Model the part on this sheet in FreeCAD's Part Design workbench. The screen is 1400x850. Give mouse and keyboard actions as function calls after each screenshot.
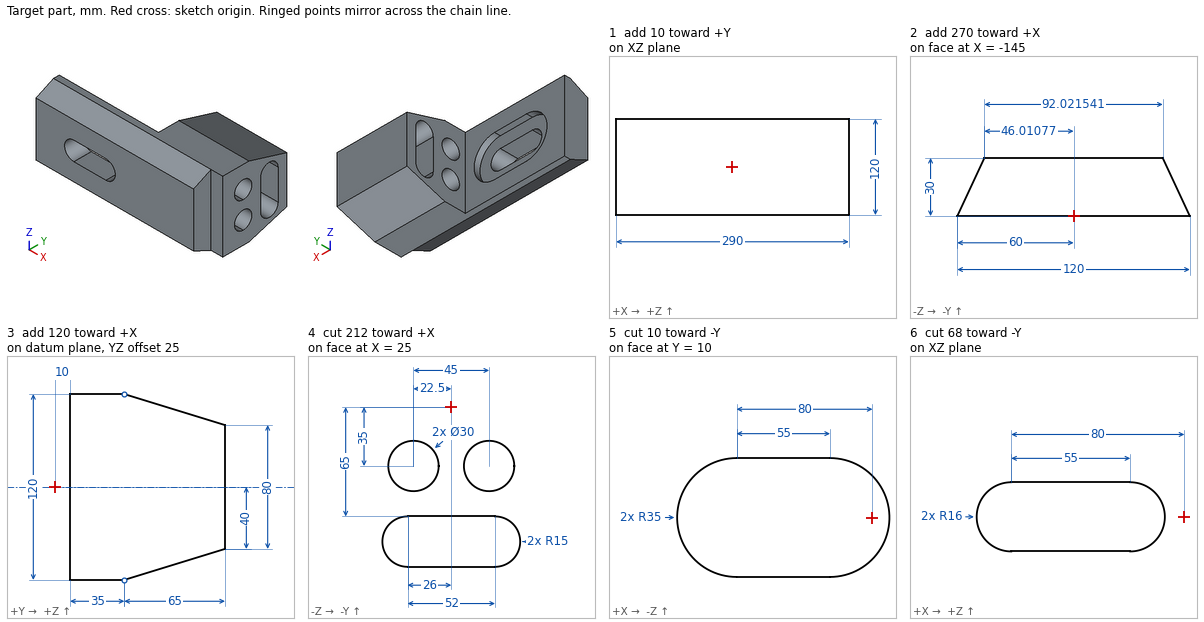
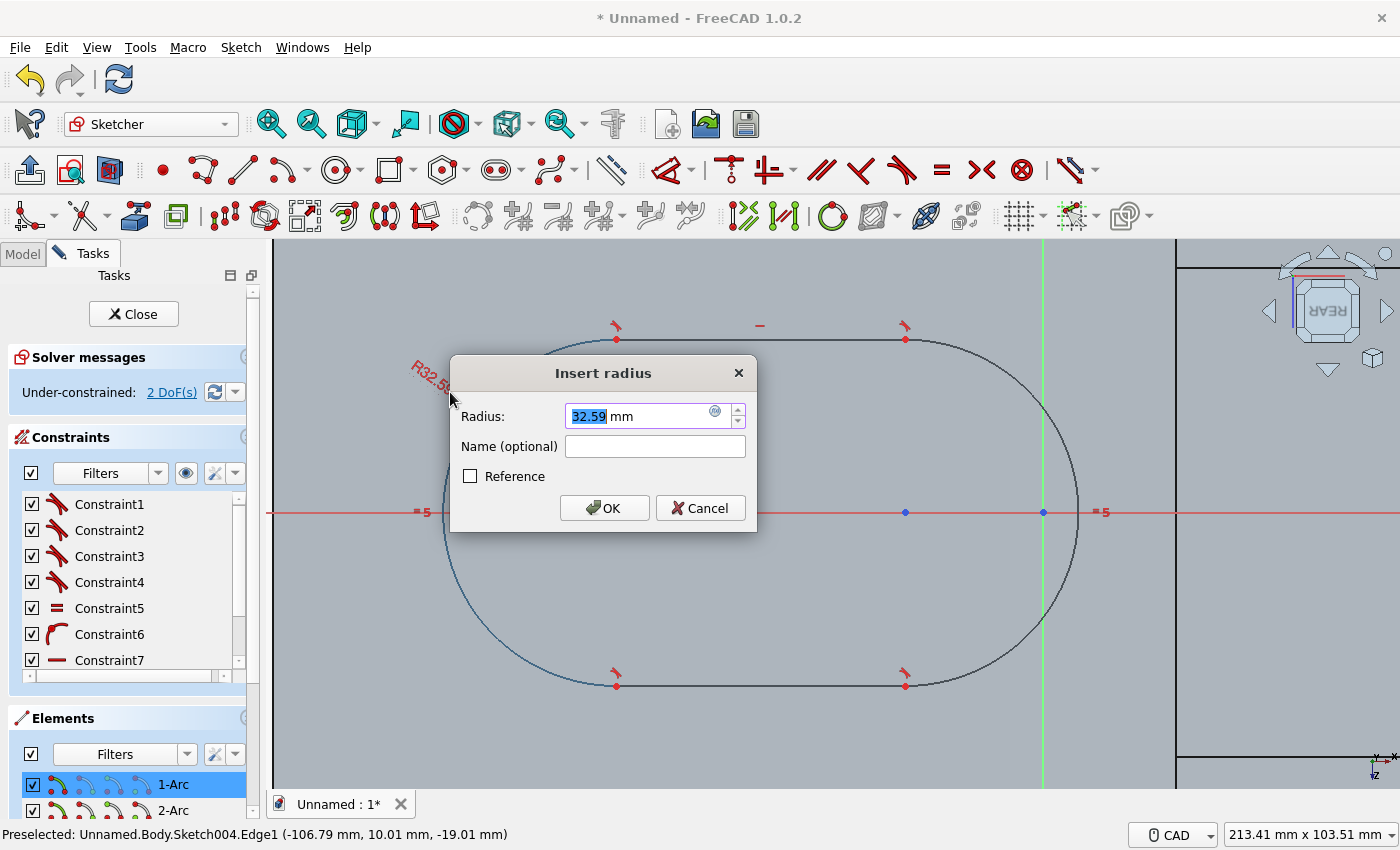
text(35)
key(Return)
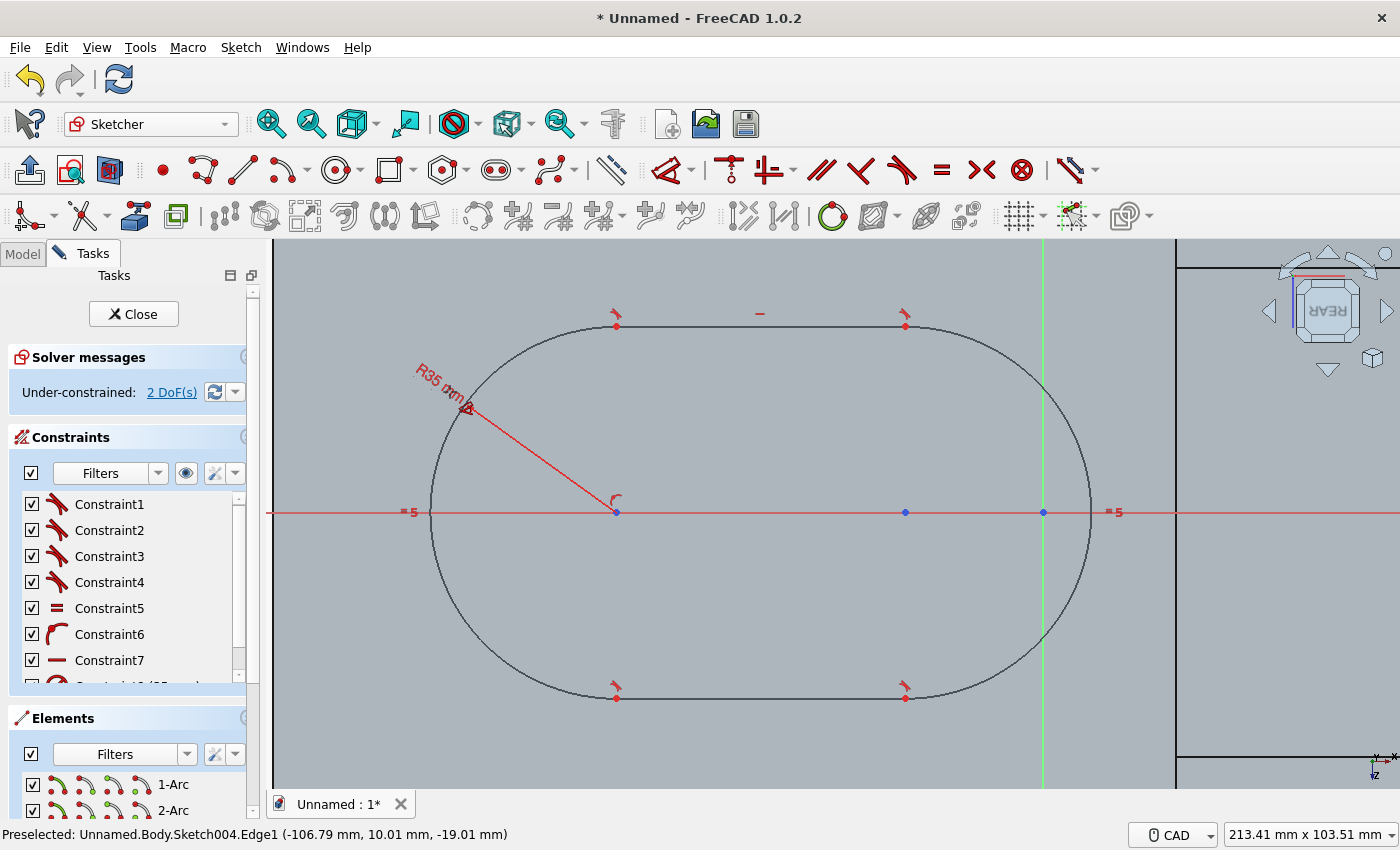
click(703, 327)
click(761, 293)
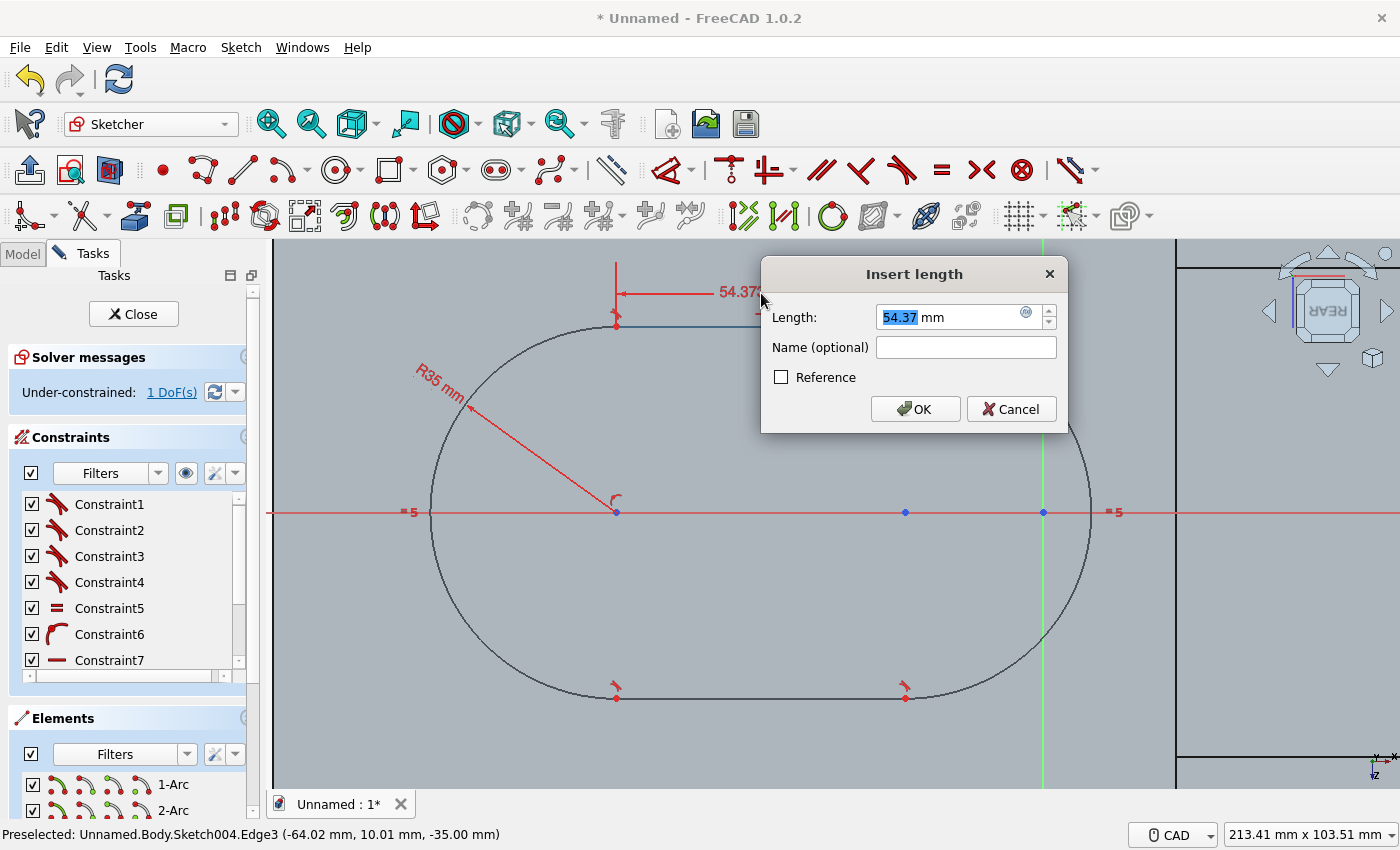
text(55)
key(Return)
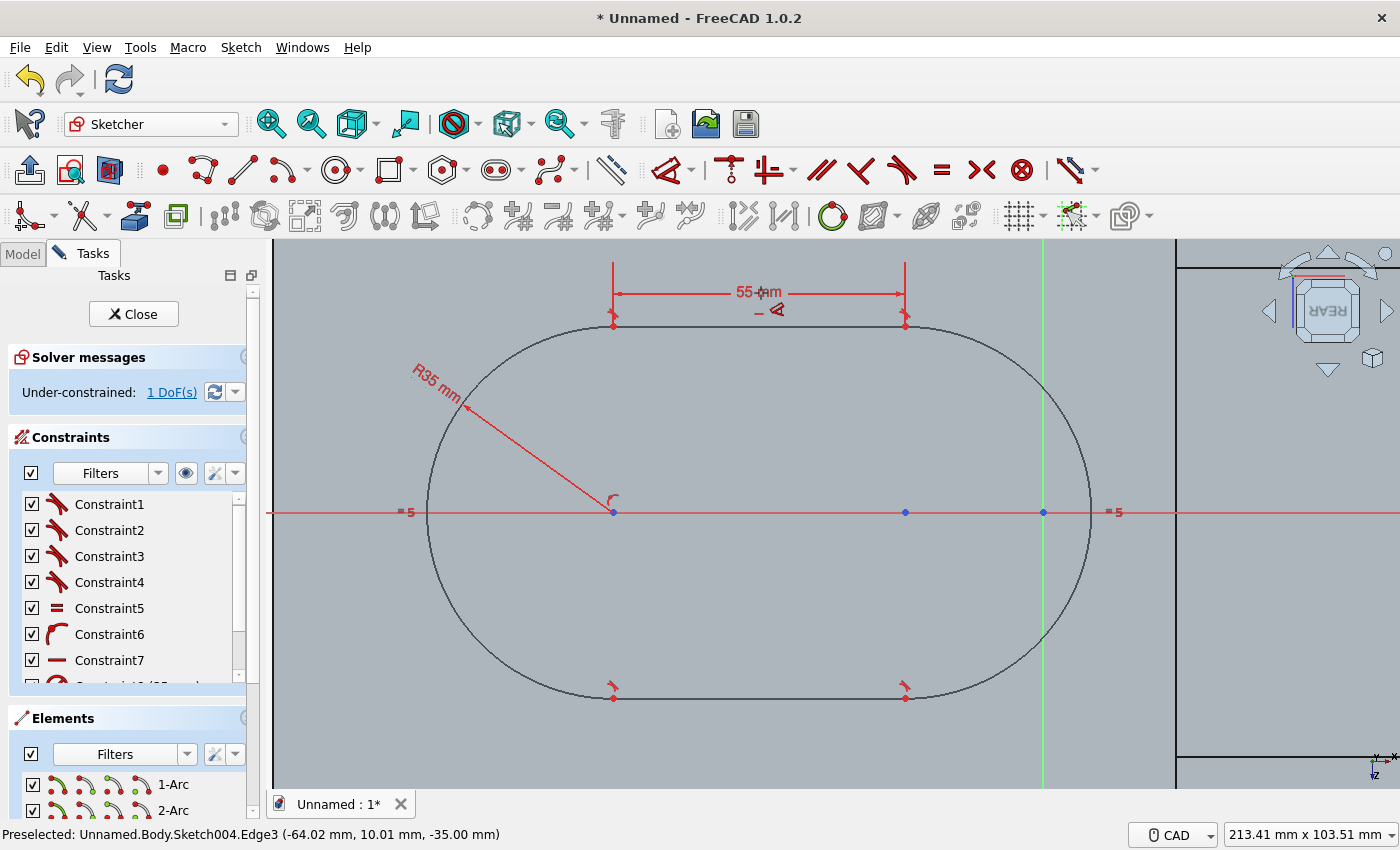
click(613, 327)
click(927, 293)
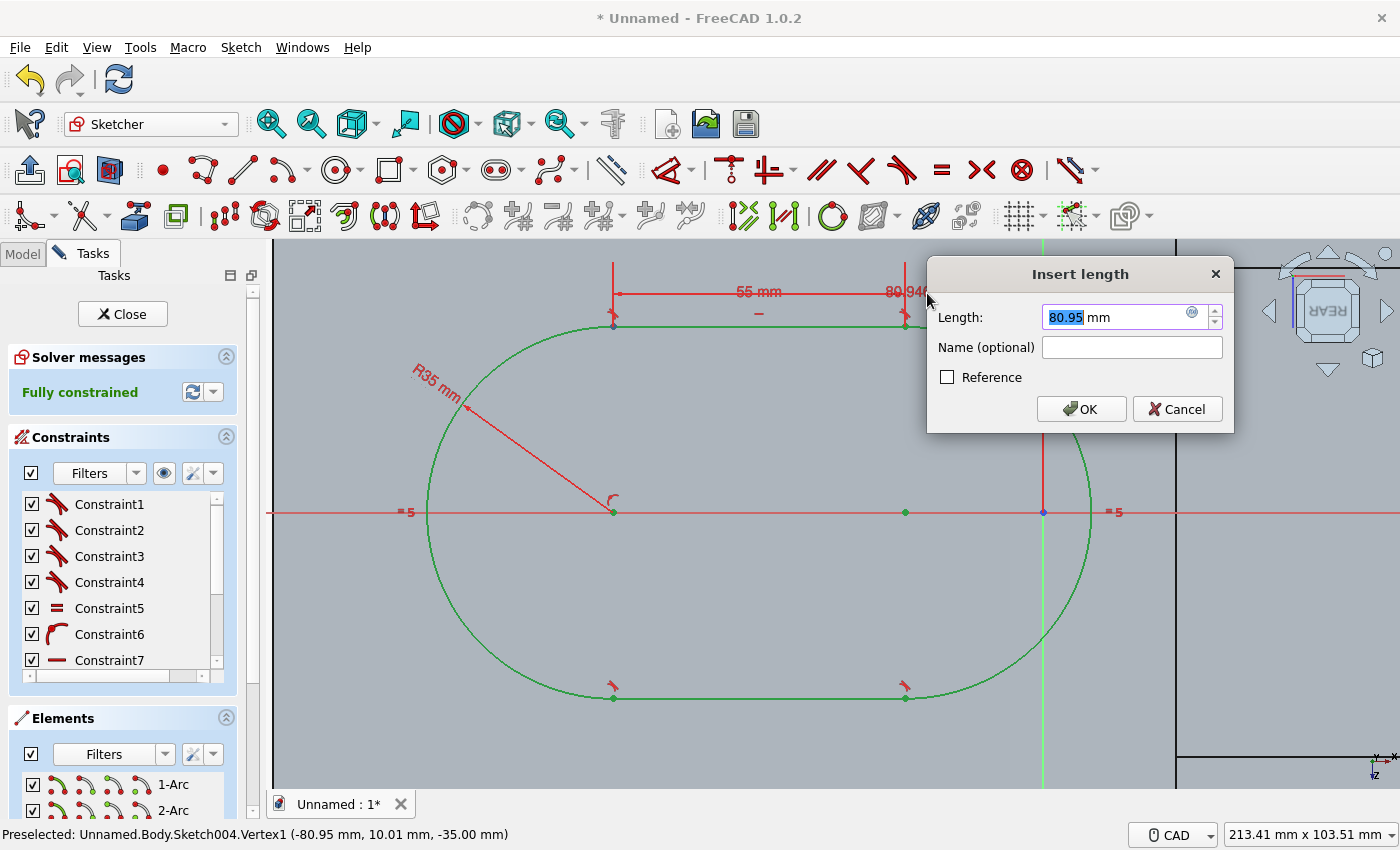
text(80)
key(Return)
key(Escape)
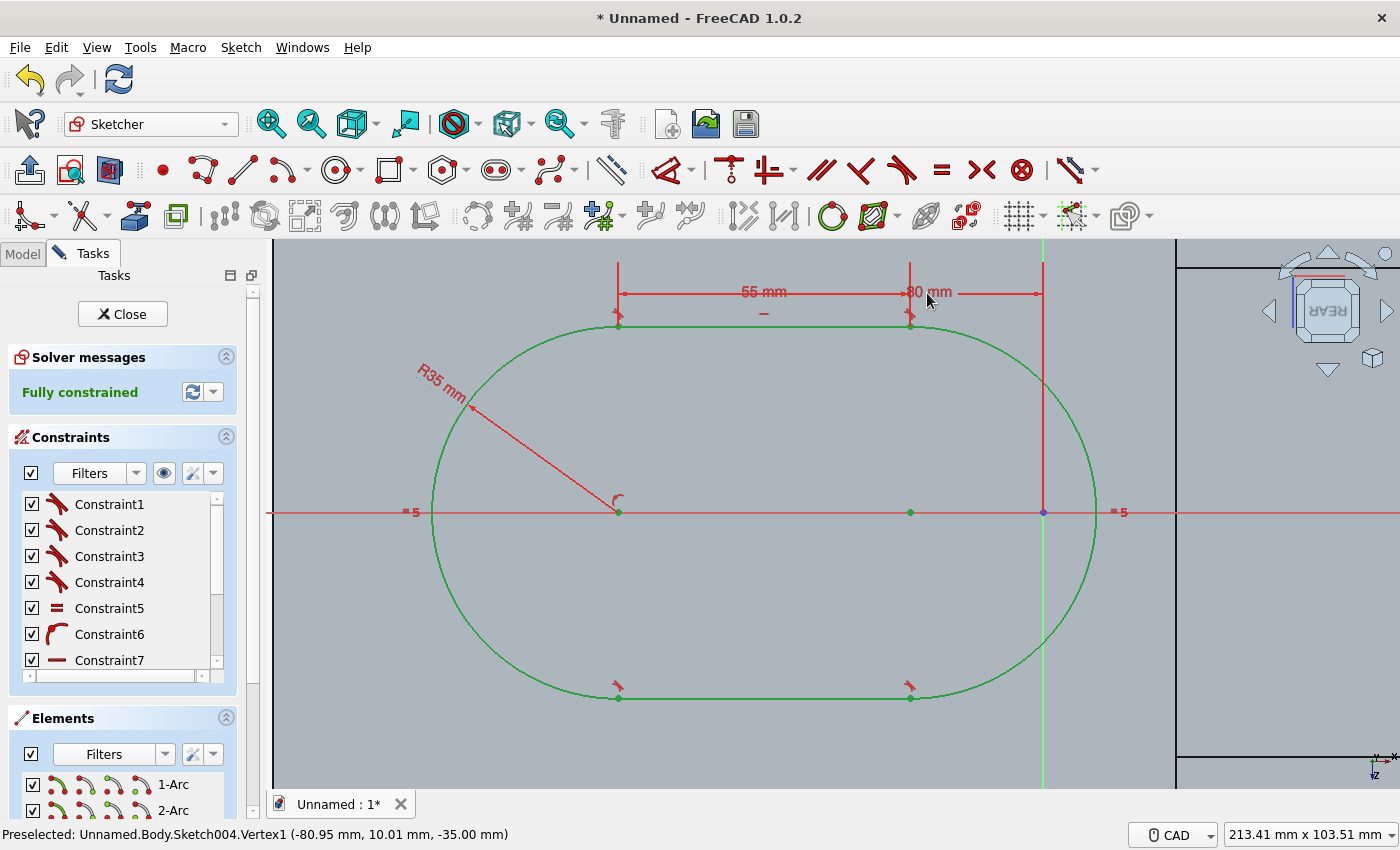
click(123, 314)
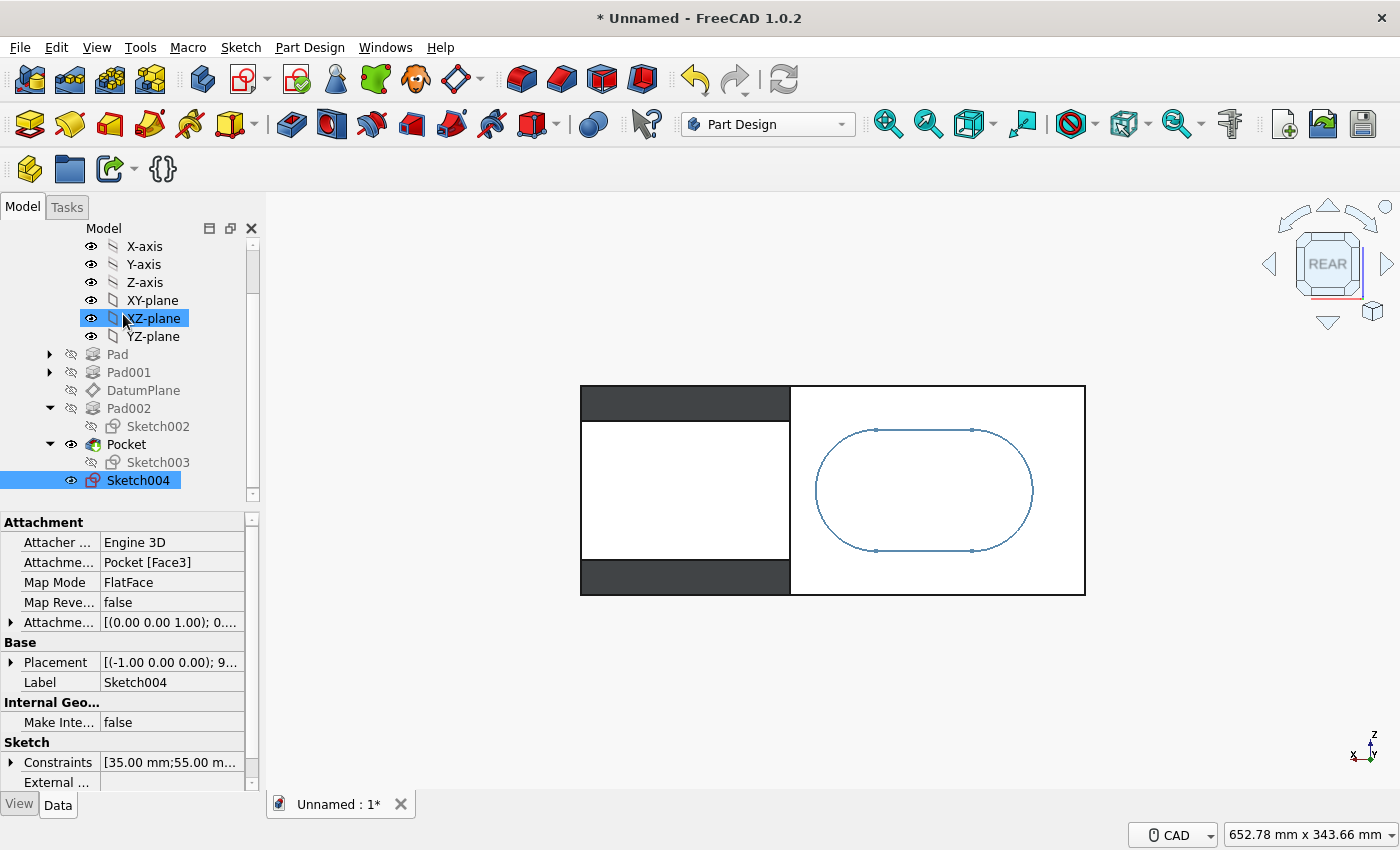
click(292, 124)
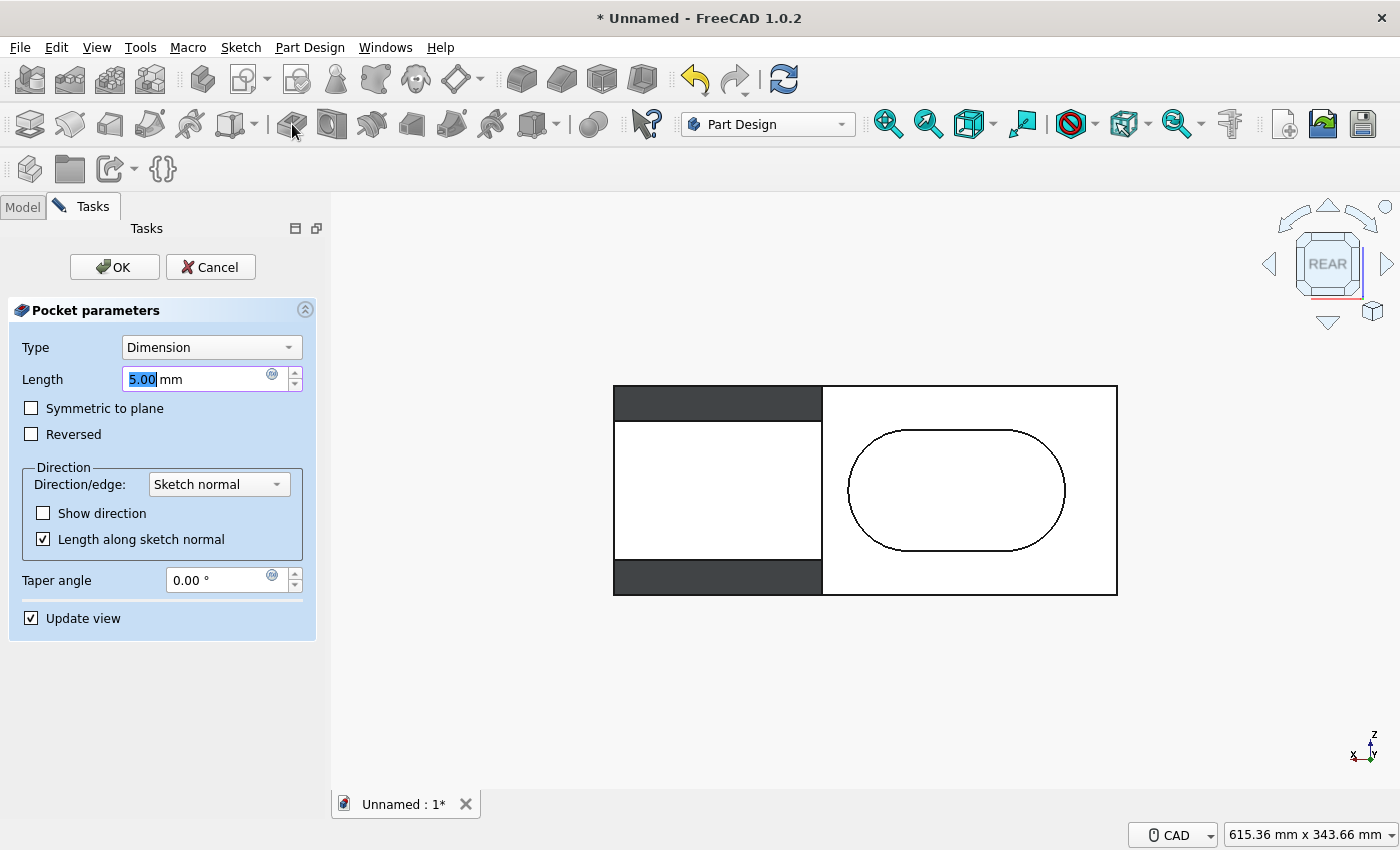
text(10)
key(Tab)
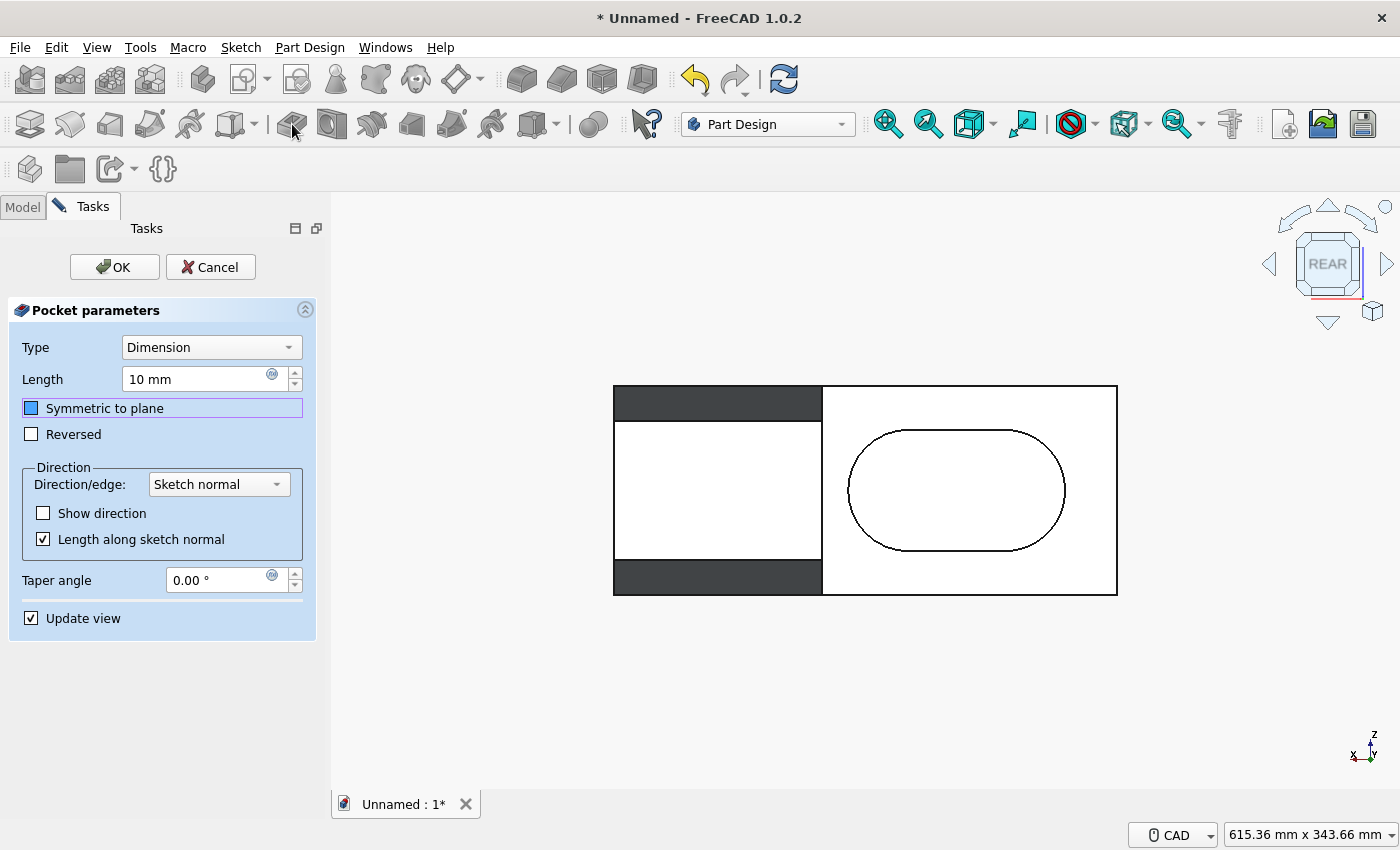
click(115, 267)